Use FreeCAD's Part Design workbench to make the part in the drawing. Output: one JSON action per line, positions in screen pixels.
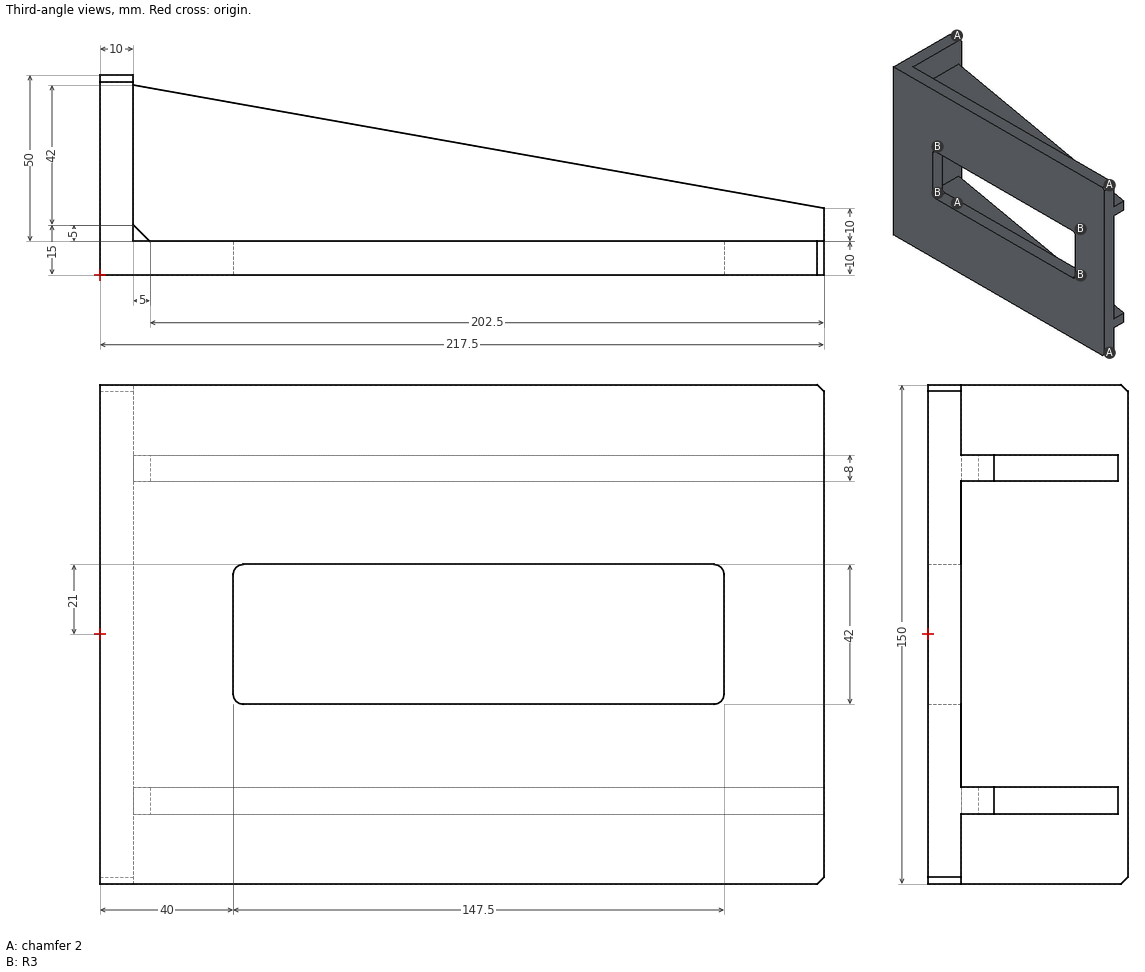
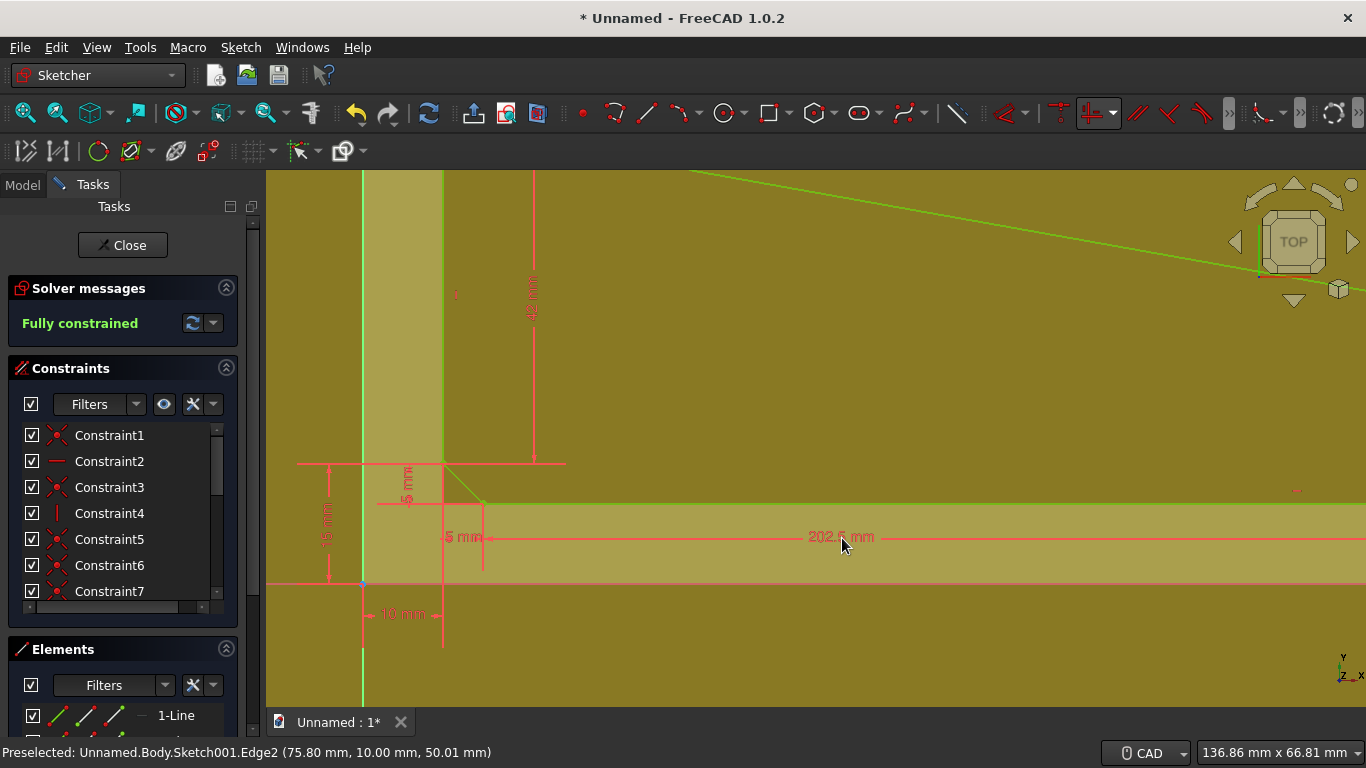
{"action": "left_click", "coordinate": [123, 245]}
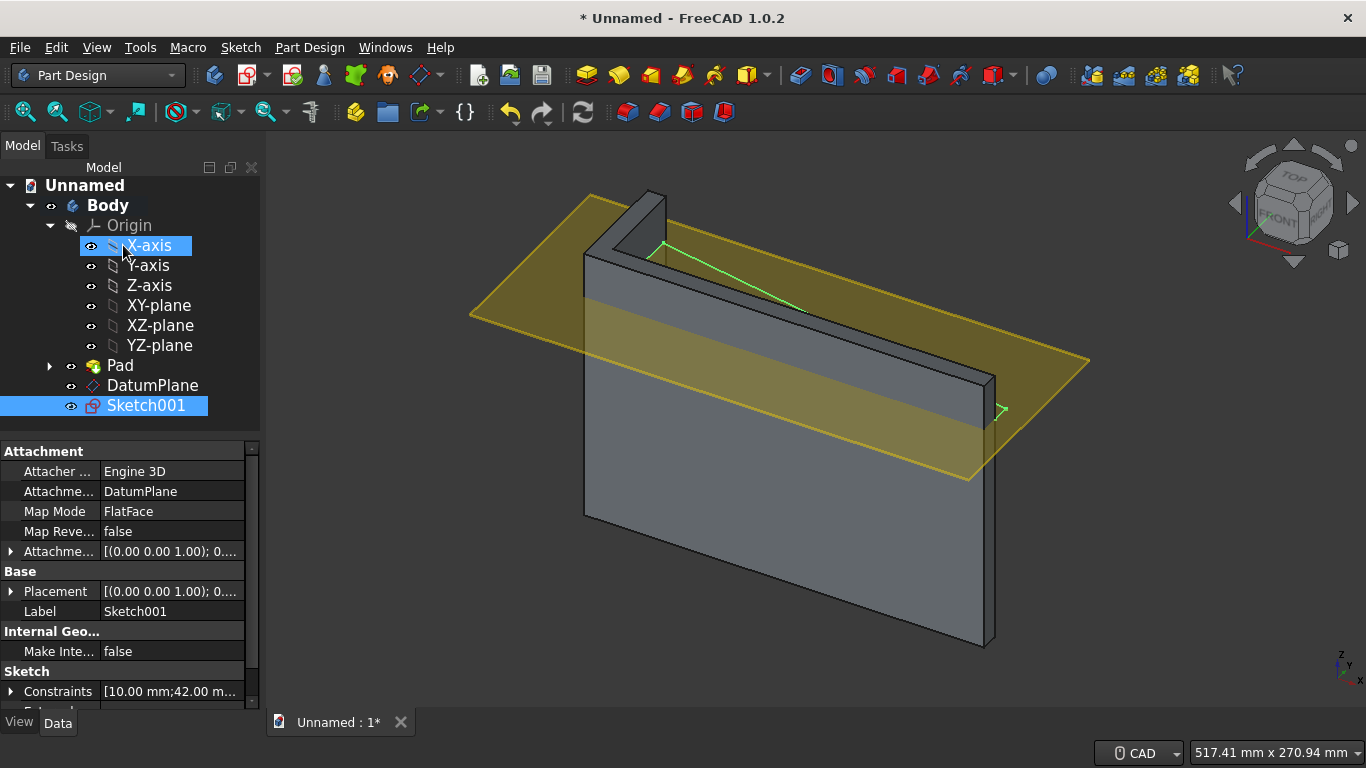
{"action": "left_click", "coordinate": [588, 76]}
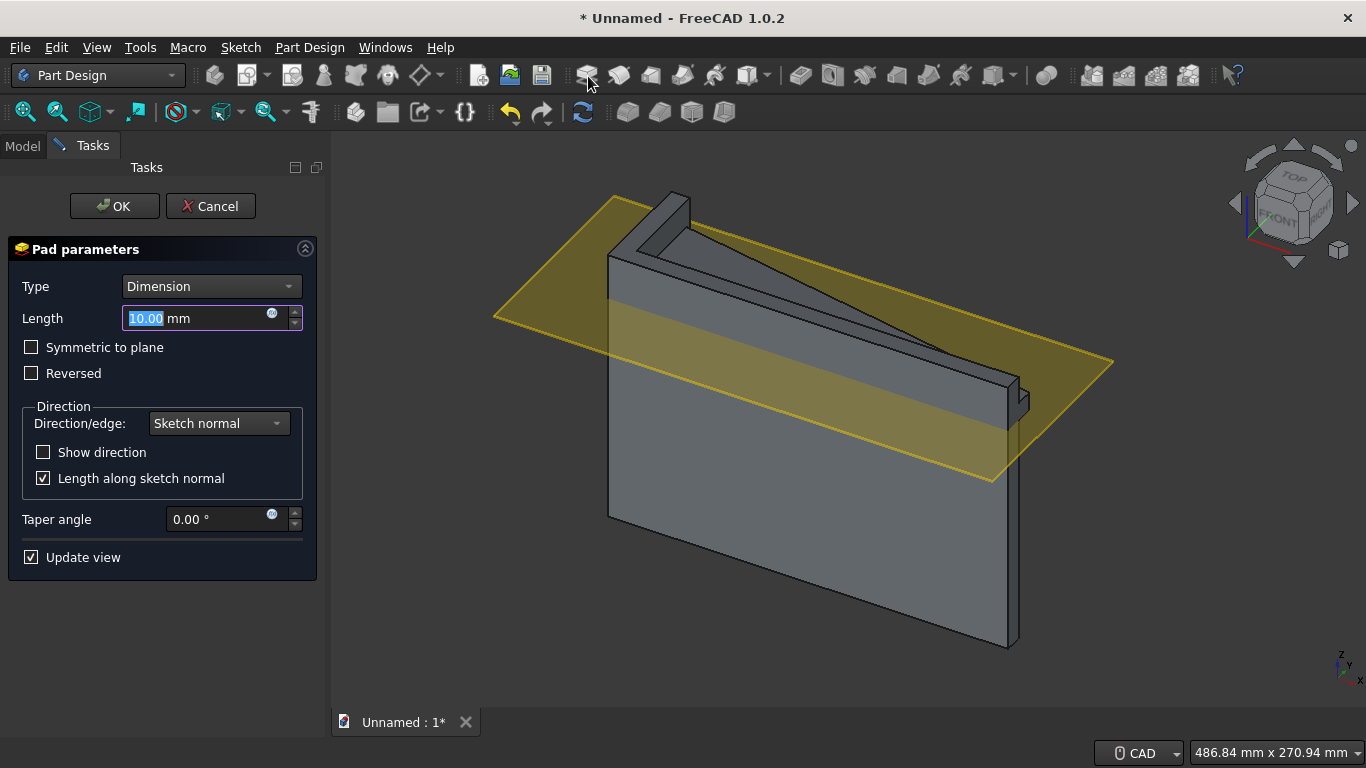
{"action": "type", "text": "8"}
{"action": "key", "text": "Tab"}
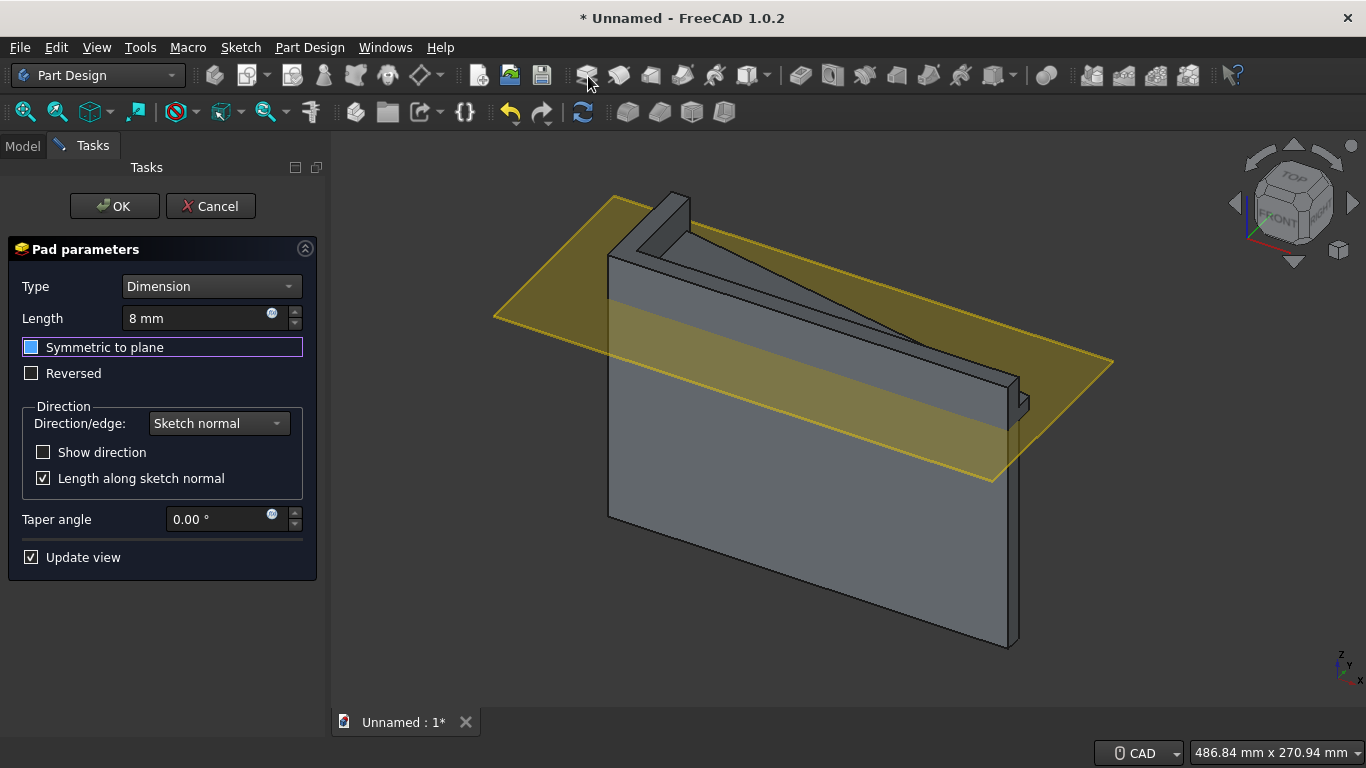
{"action": "left_click", "coordinate": [30, 347]}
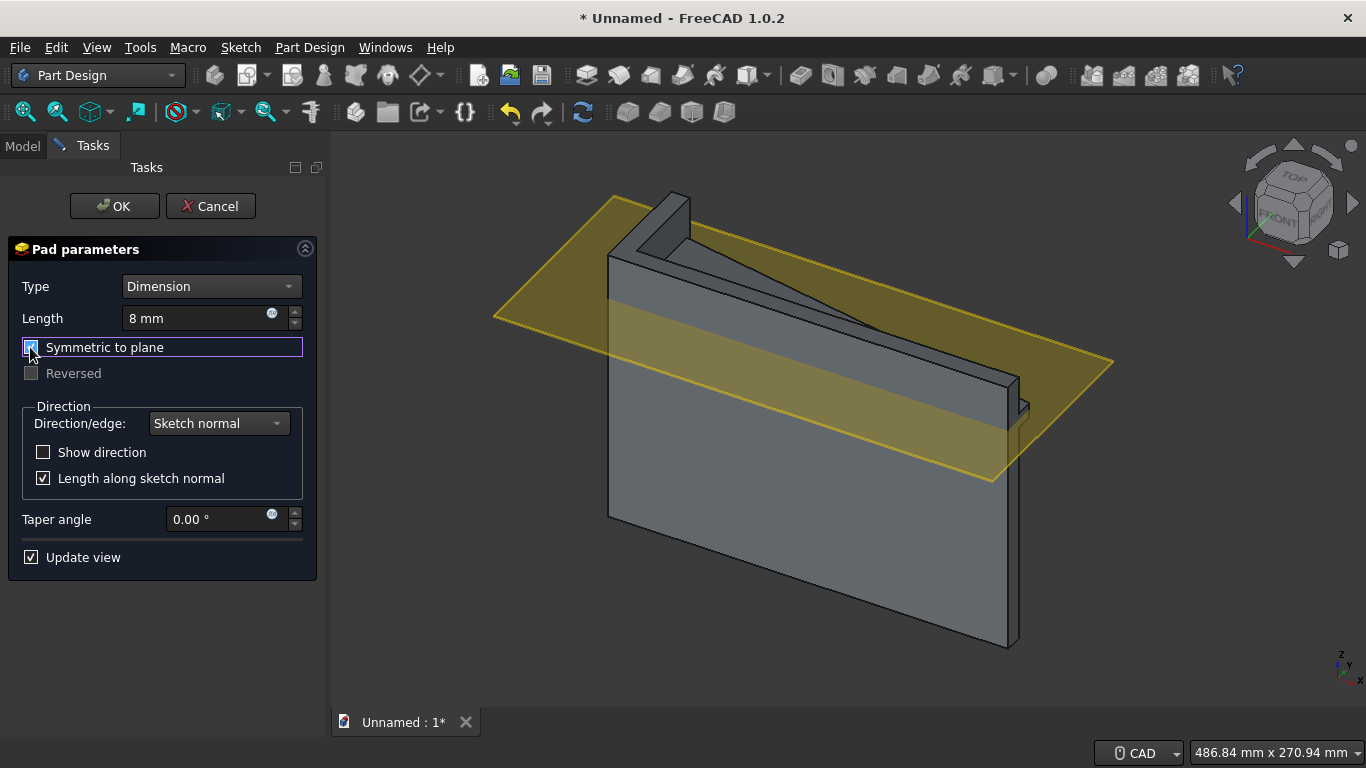
{"action": "left_click", "coordinate": [115, 206]}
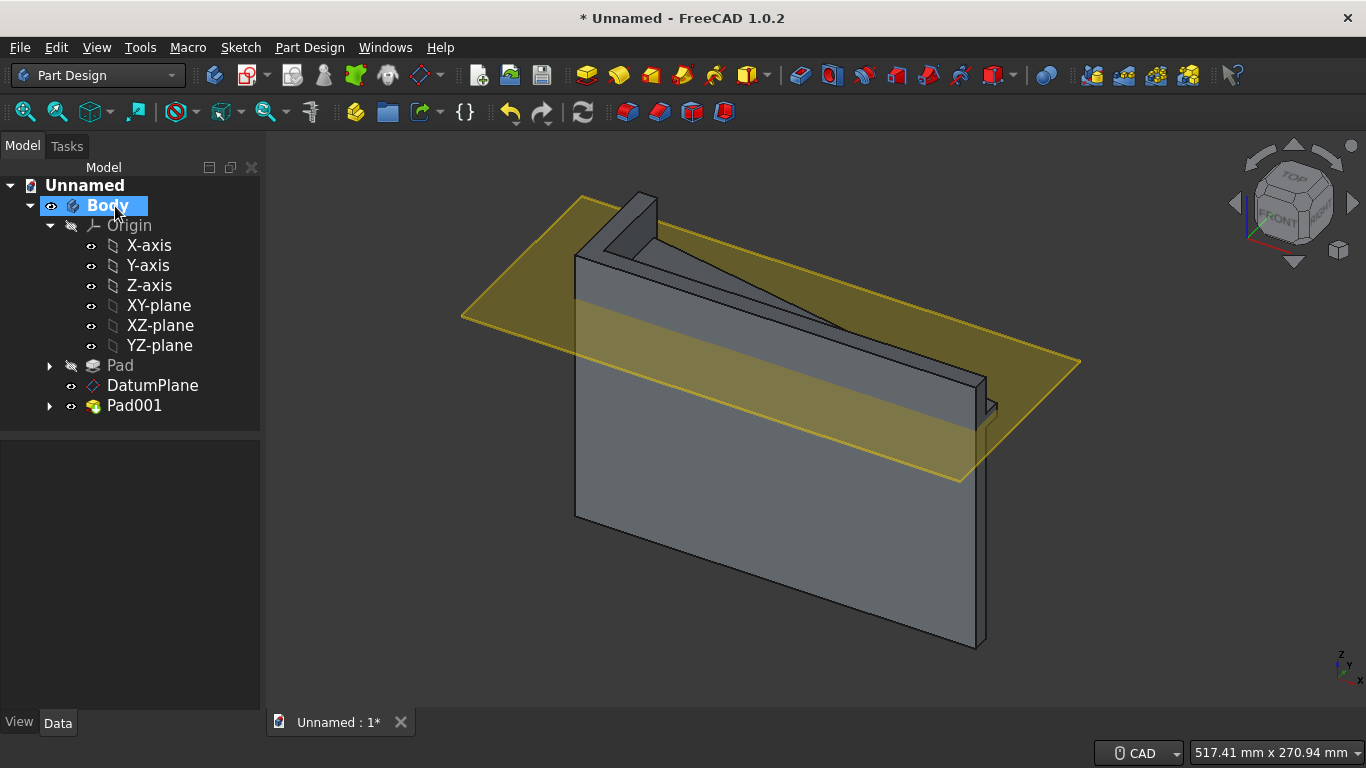
{"action": "left_click", "coordinate": [116, 386]}
{"action": "key", "text": "space"}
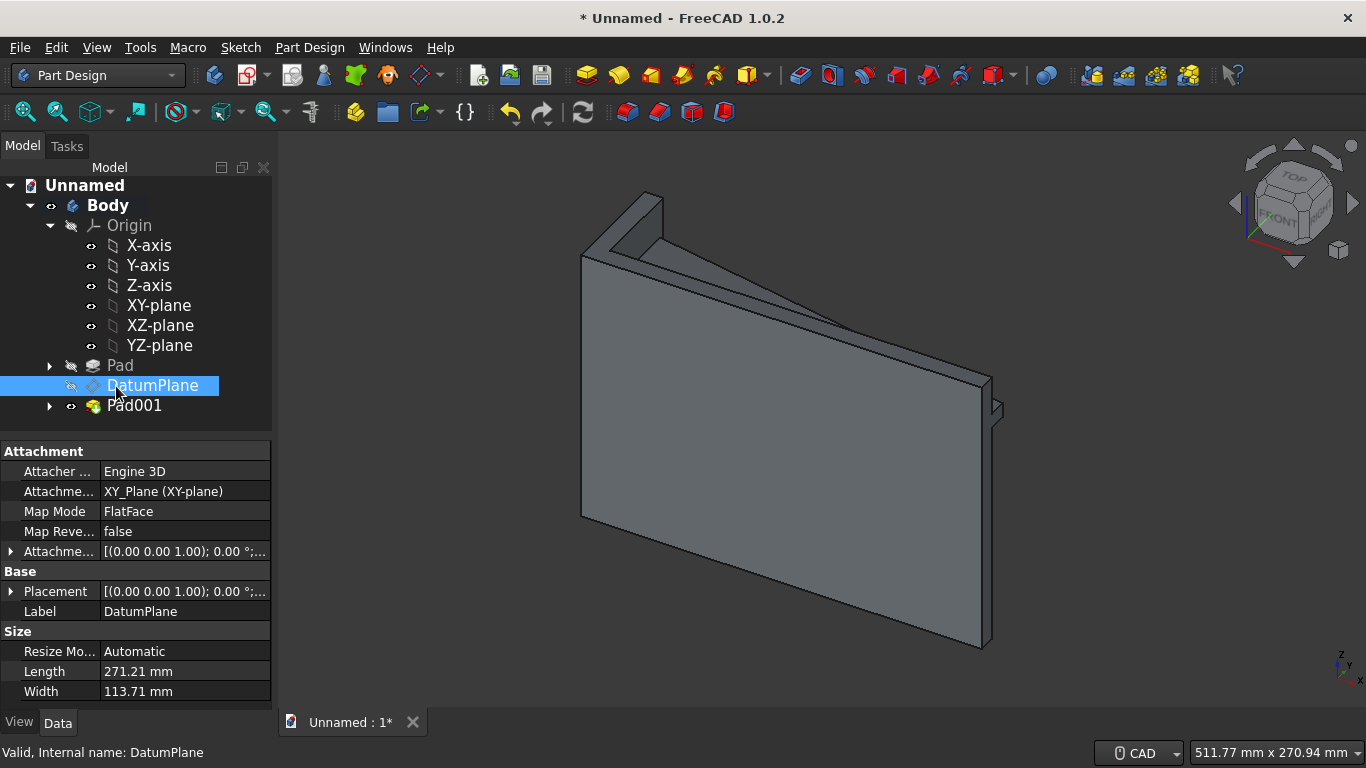
{"action": "left_click", "coordinate": [987, 381]}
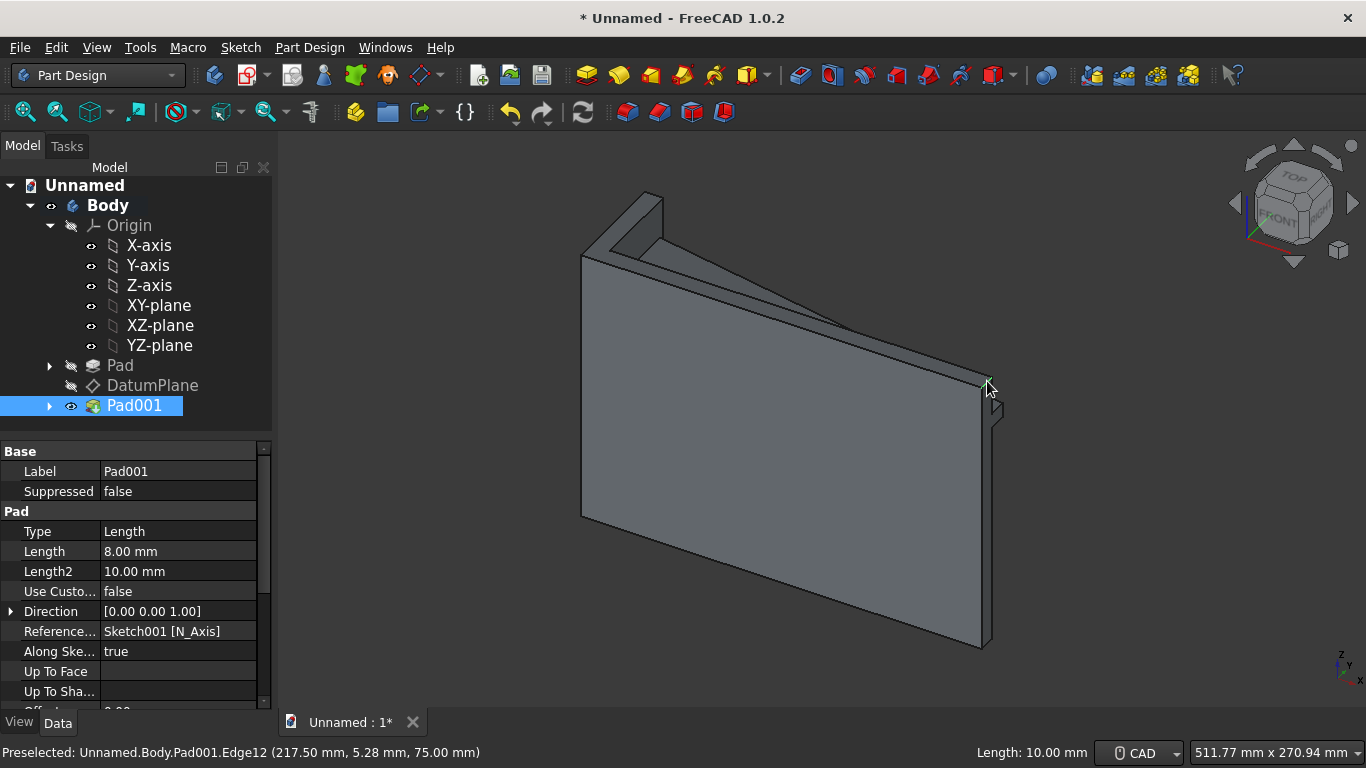
{"action": "scroll", "coordinate": [654, 194], "scroll_direction": "up", "scroll_amount": 4}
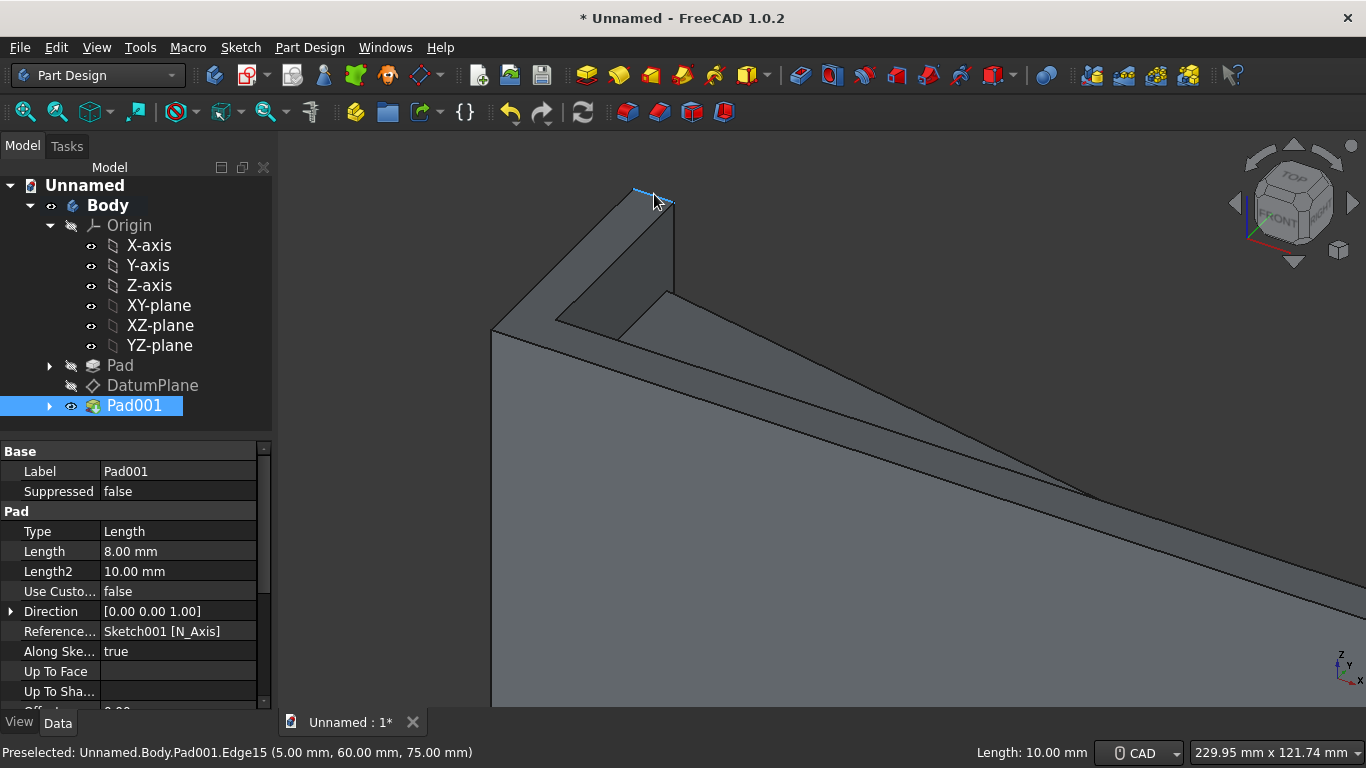
{"action": "left_click", "coordinate": [26, 112]}